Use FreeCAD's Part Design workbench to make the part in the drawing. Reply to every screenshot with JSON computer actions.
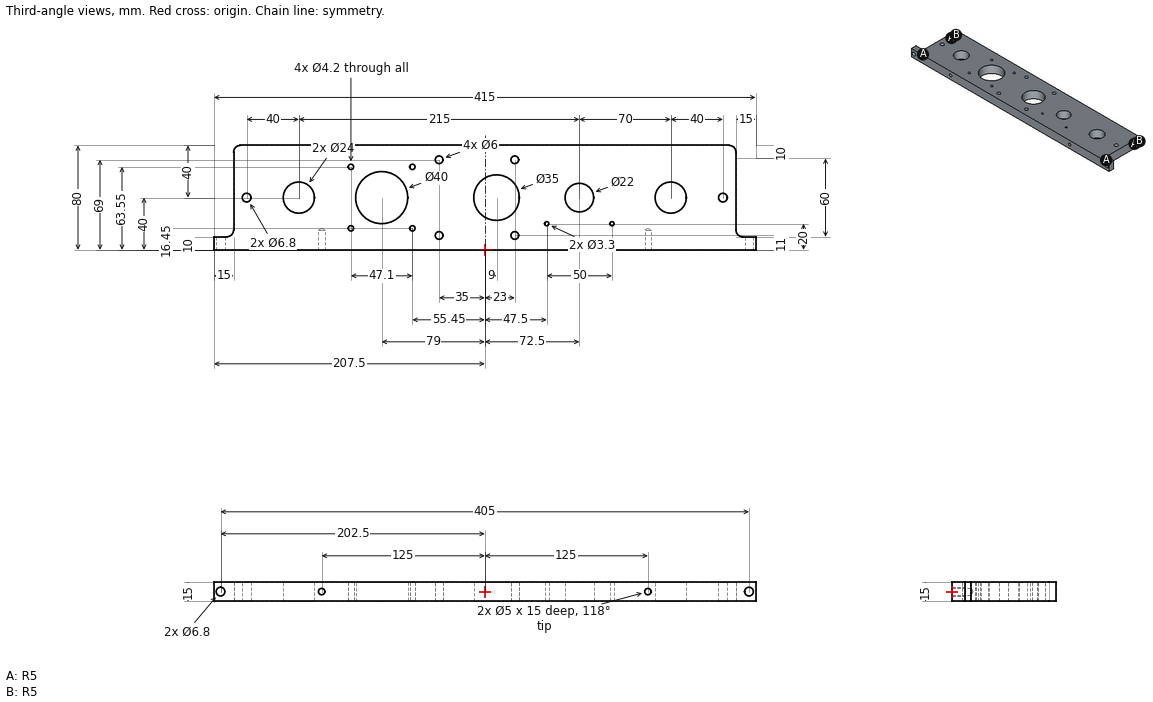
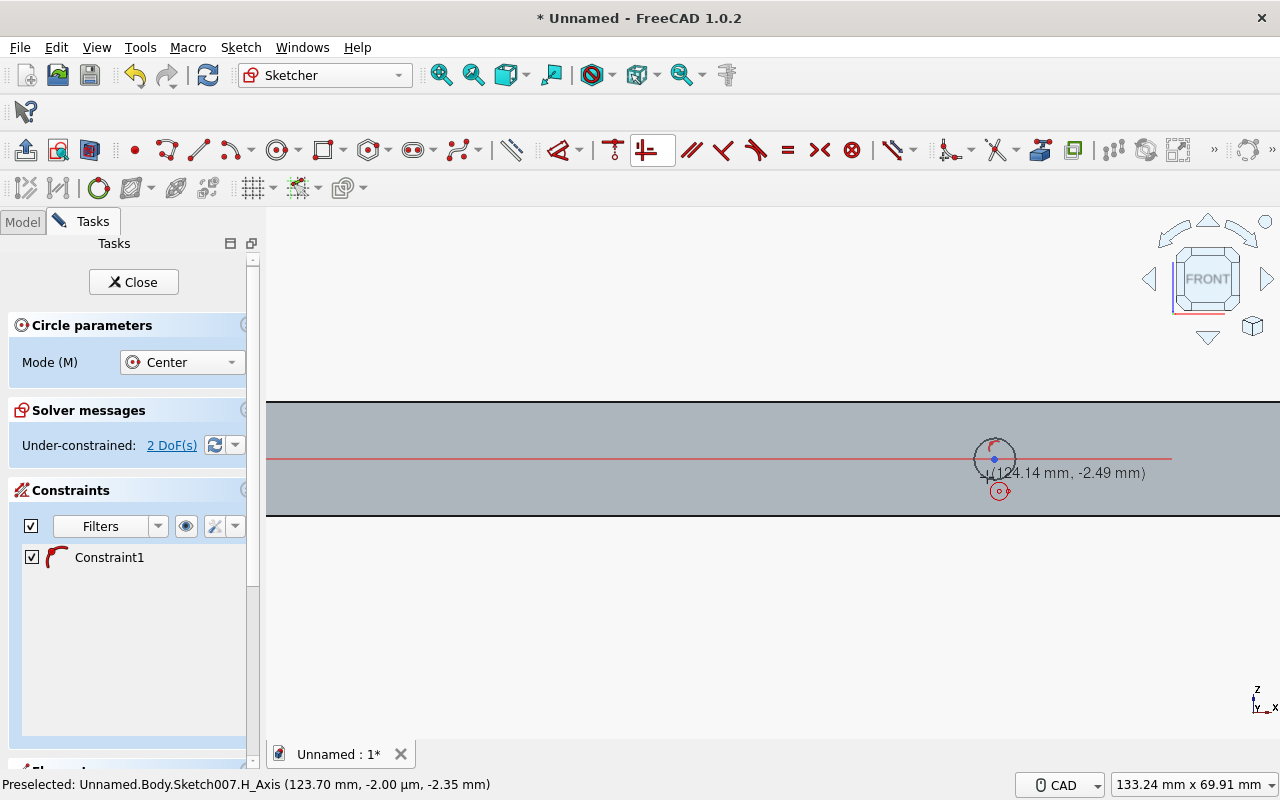
{"action": "scroll", "coordinate": [990, 479], "scroll_direction": "down", "scroll_amount": 6}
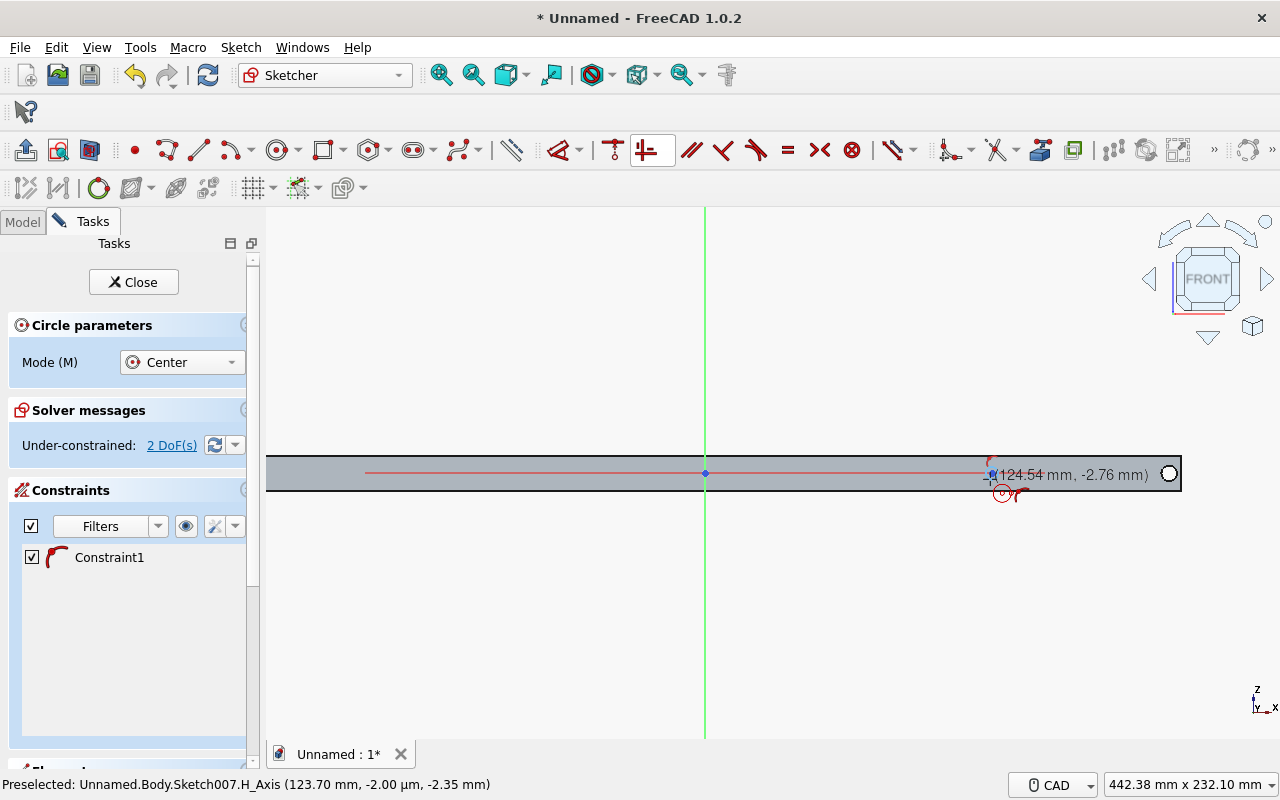
{"action": "scroll", "coordinate": [419, 473], "scroll_direction": "up", "scroll_amount": 7}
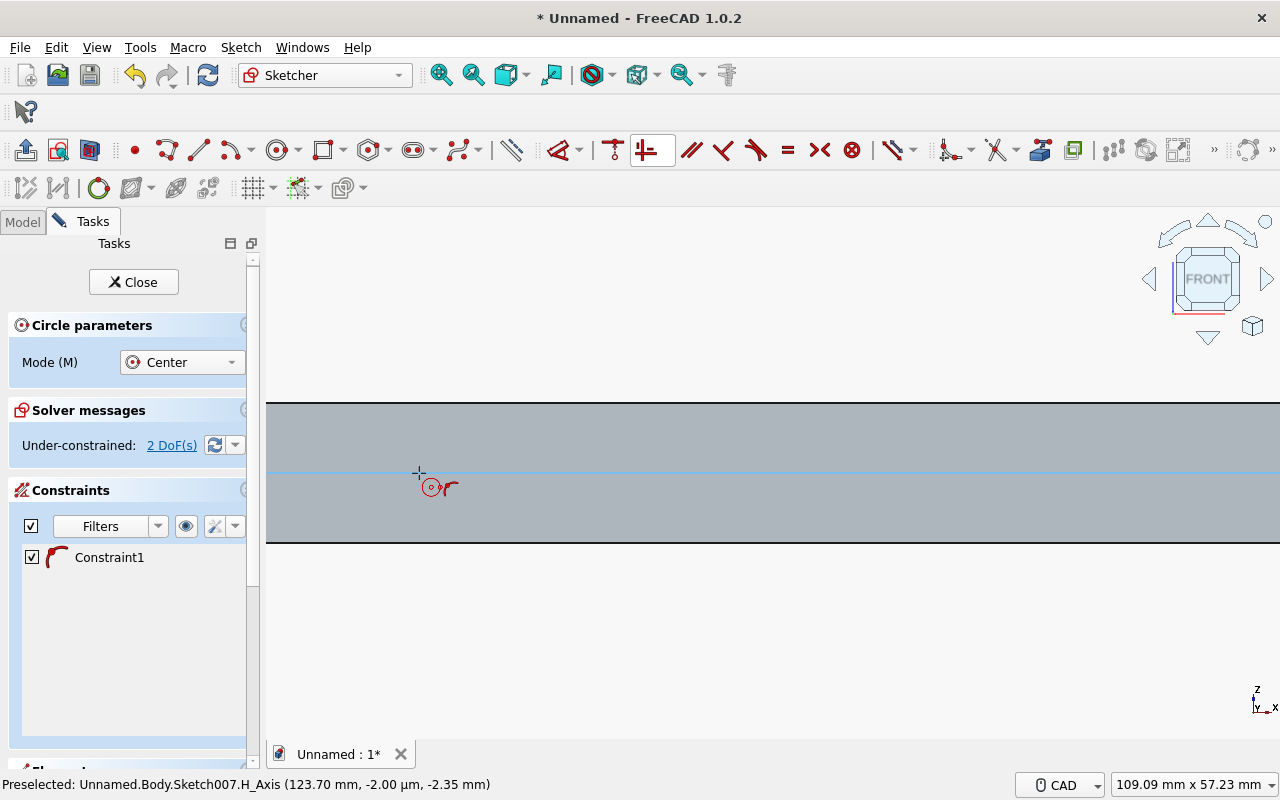
{"action": "scroll", "coordinate": [418, 473], "scroll_direction": "down", "scroll_amount": 7}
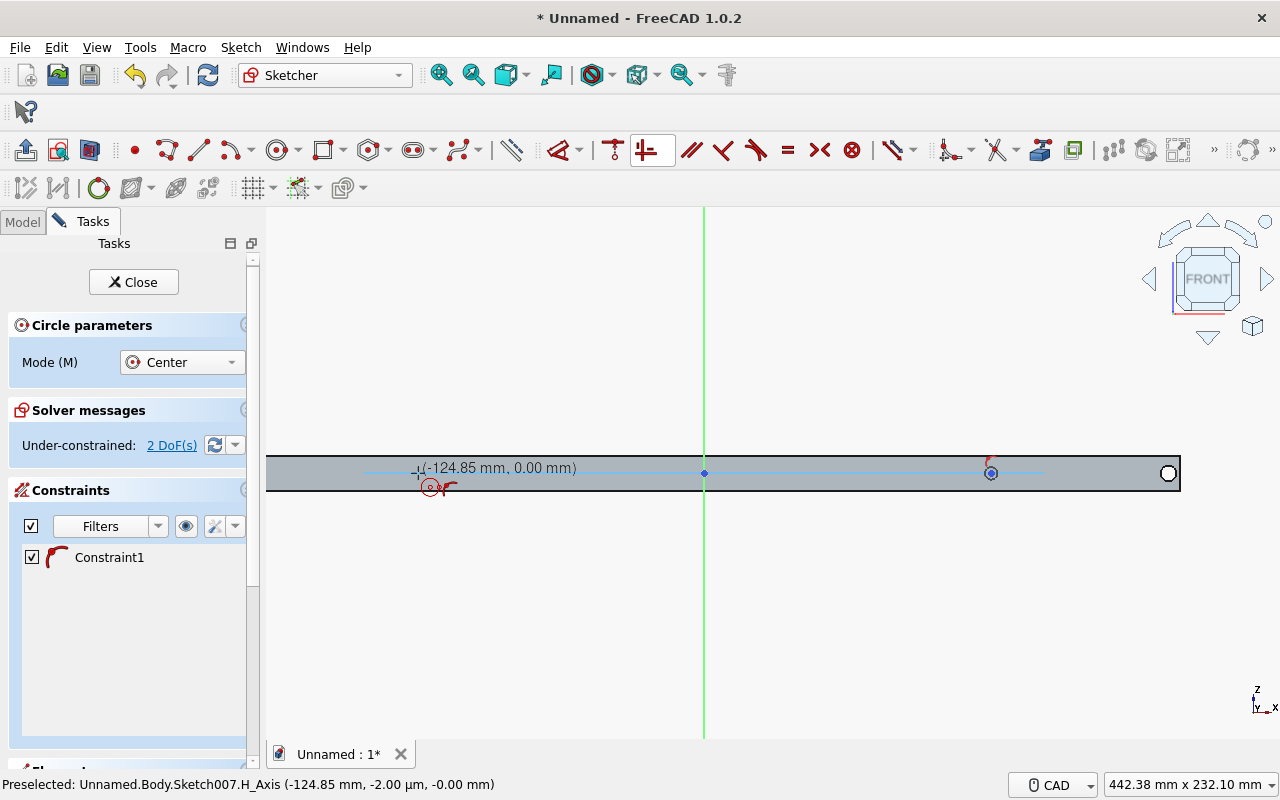
{"action": "left_click", "coordinate": [418, 473]}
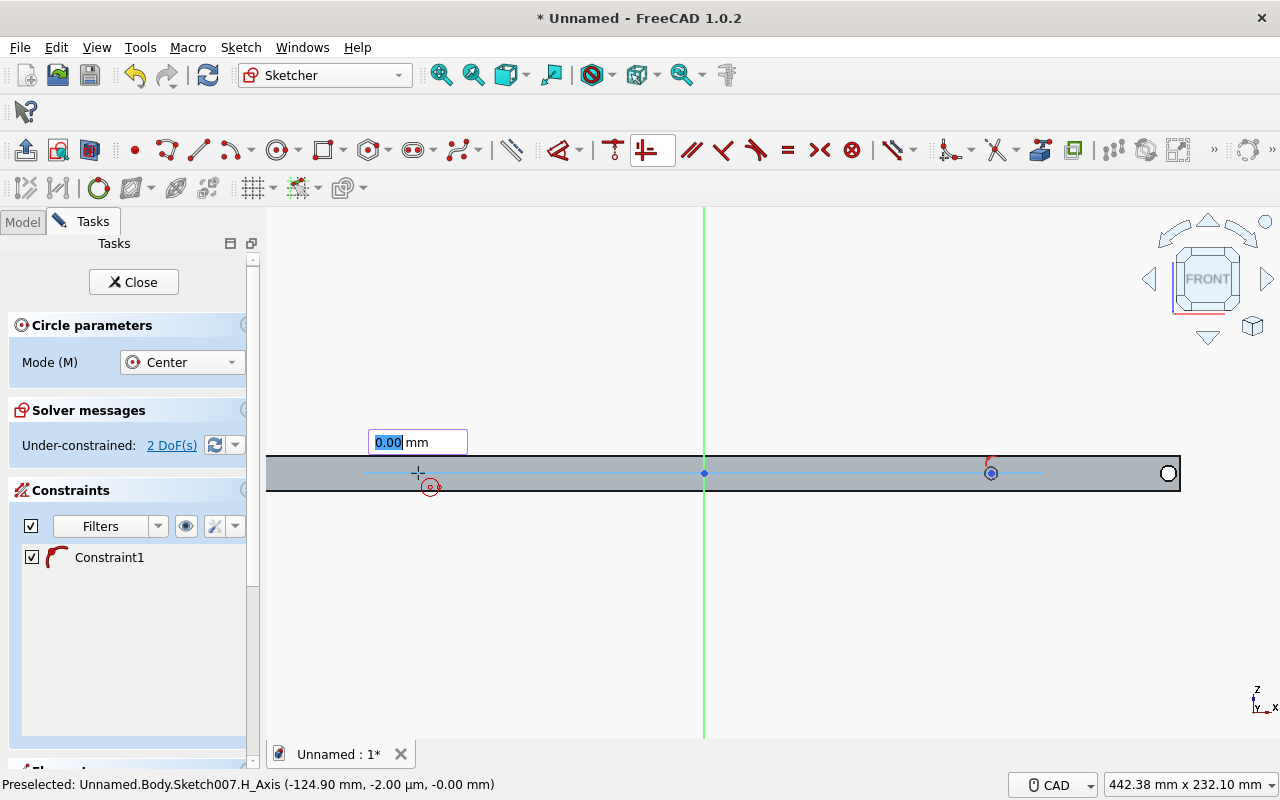
{"action": "scroll", "coordinate": [416, 479], "scroll_direction": "up", "scroll_amount": 6}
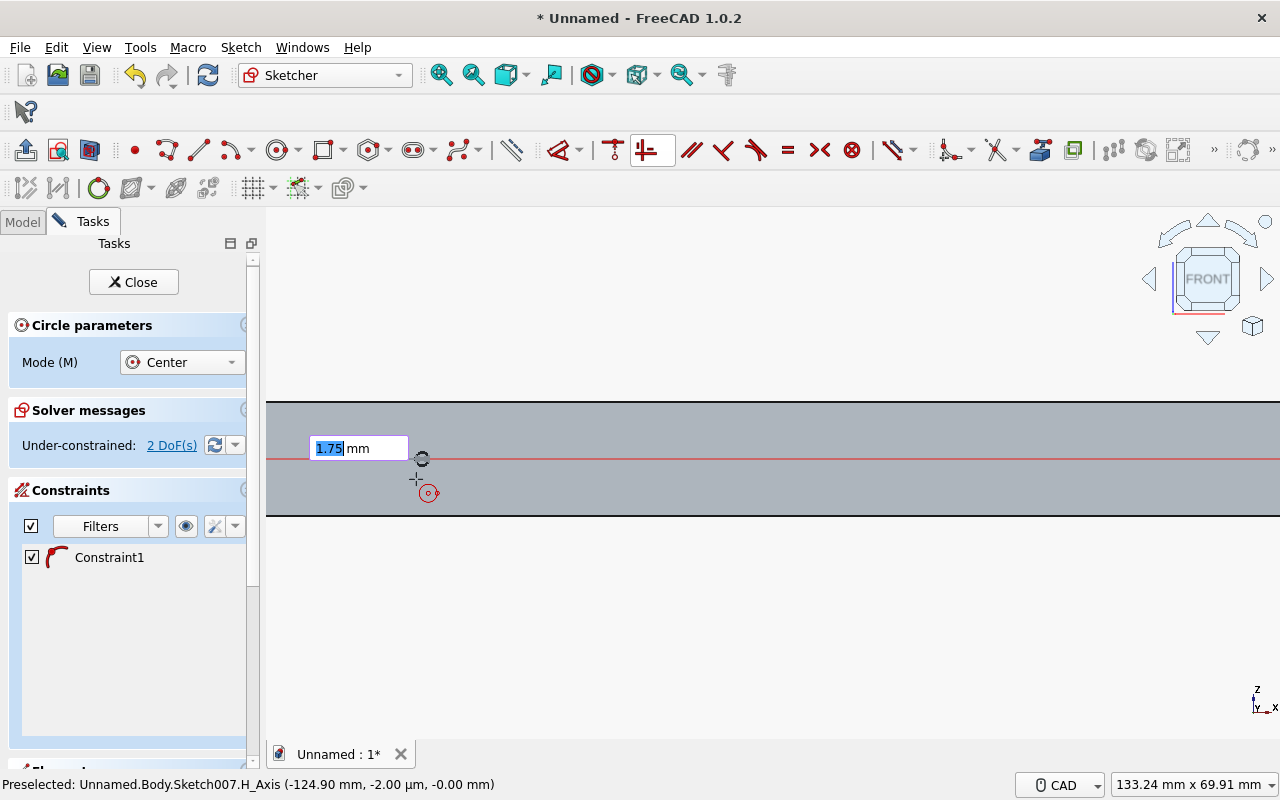
{"action": "left_click", "coordinate": [415, 477]}
{"action": "key", "text": "Escape"}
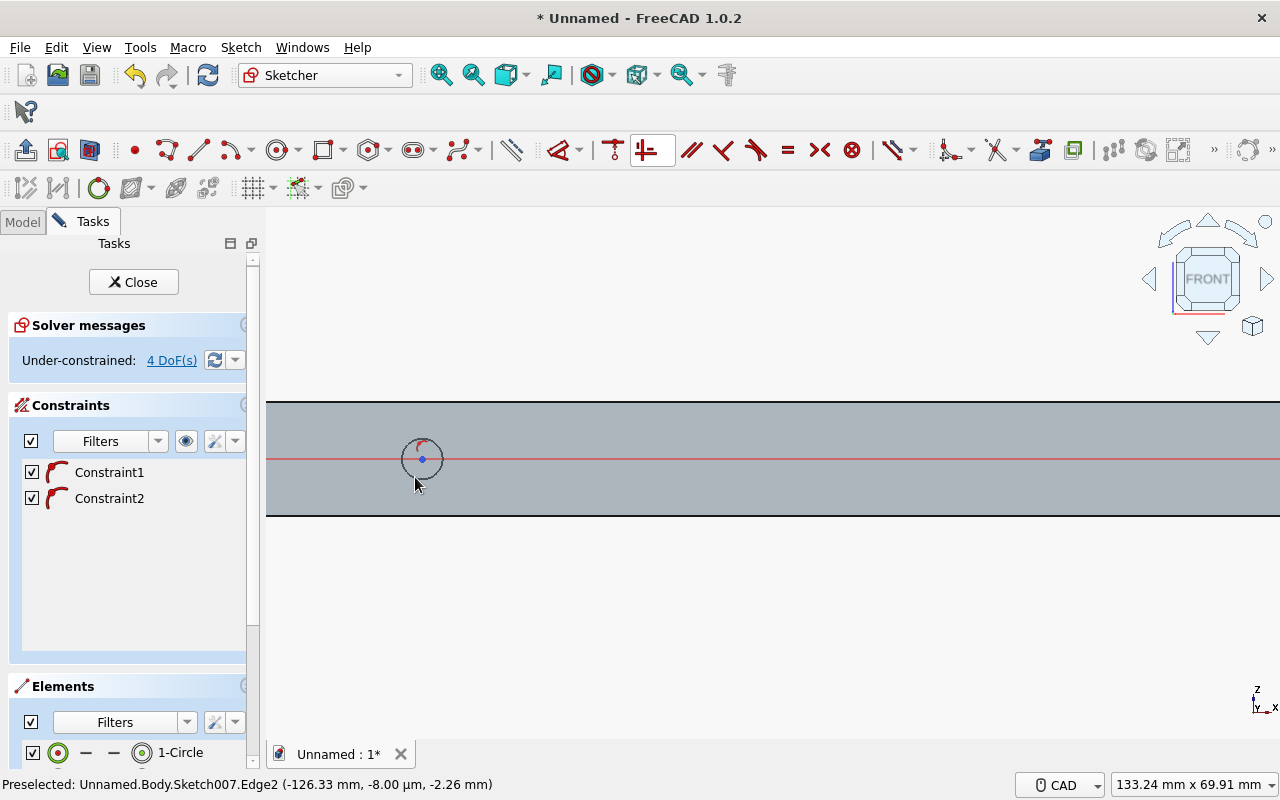
{"action": "scroll", "coordinate": [416, 479], "scroll_direction": "down", "scroll_amount": 6}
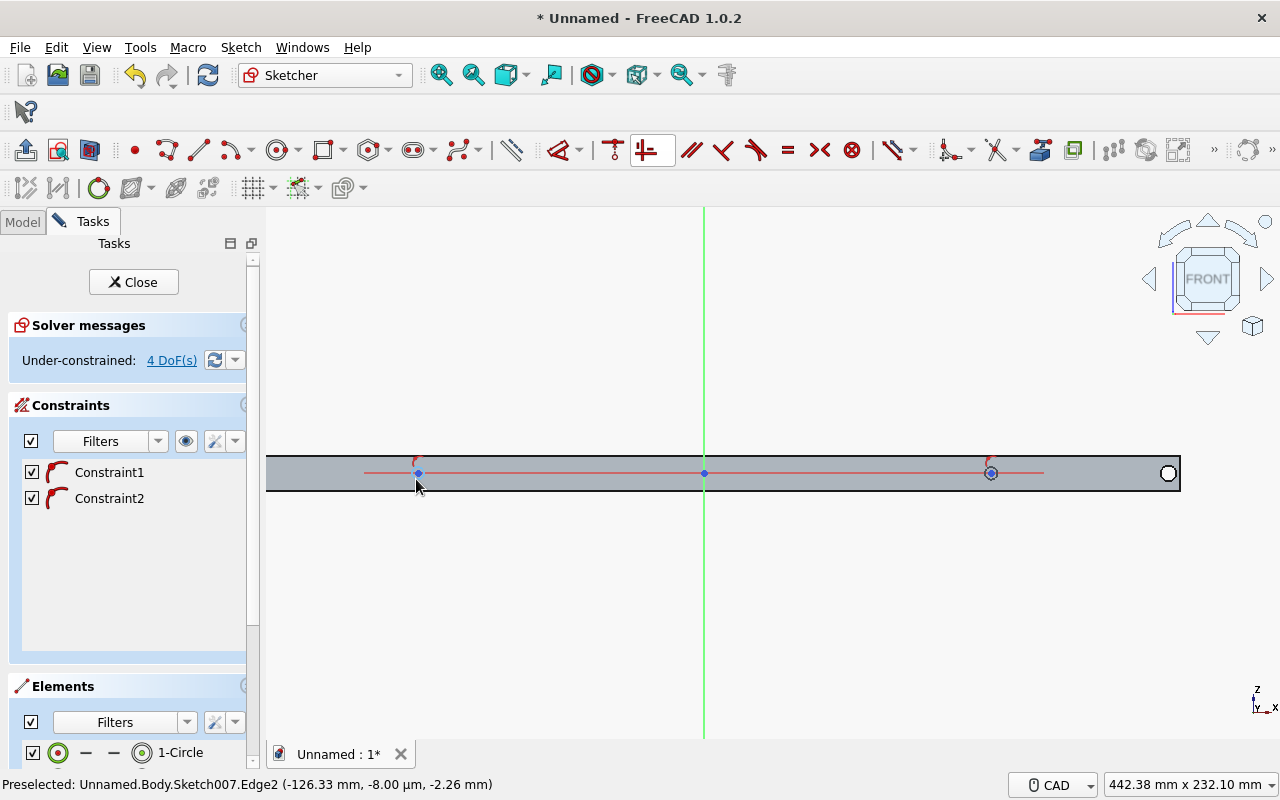
{"action": "scroll", "coordinate": [996, 469], "scroll_direction": "up", "scroll_amount": 6}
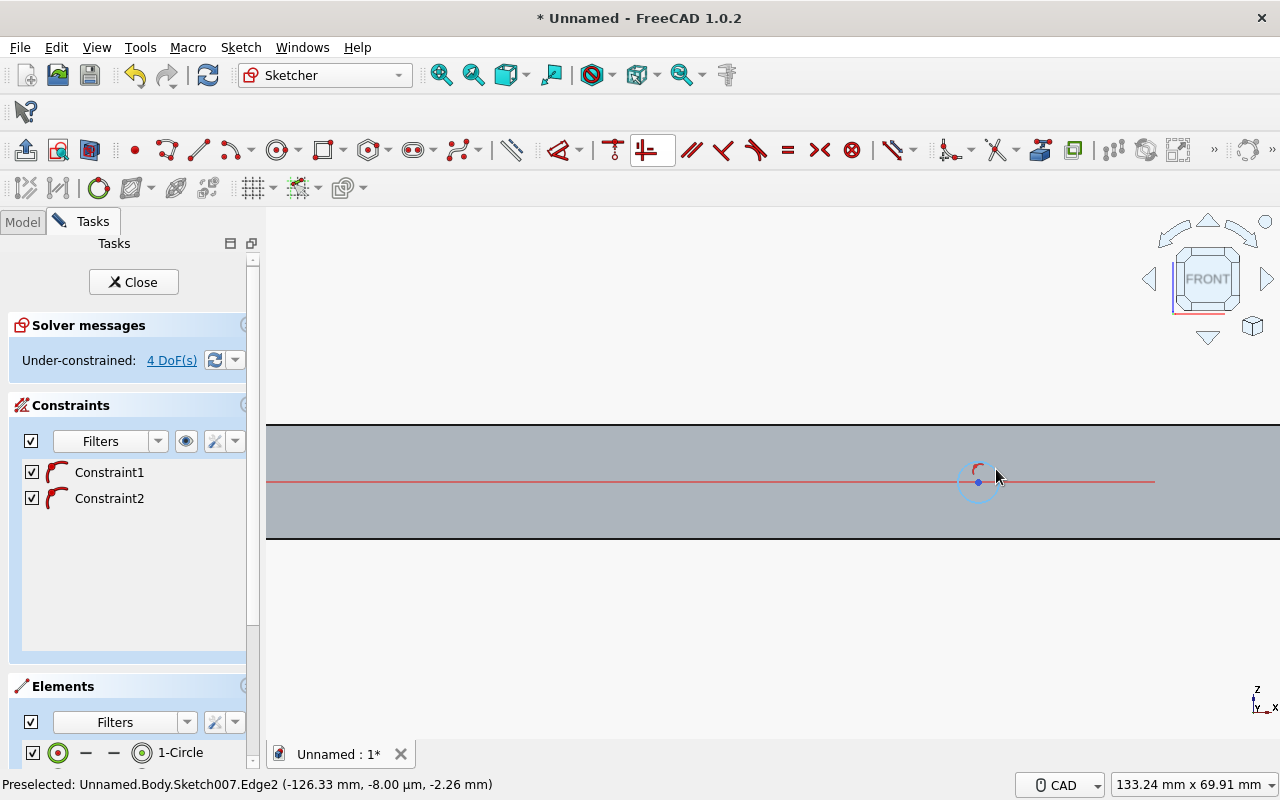
{"action": "left_click", "coordinate": [993, 468]}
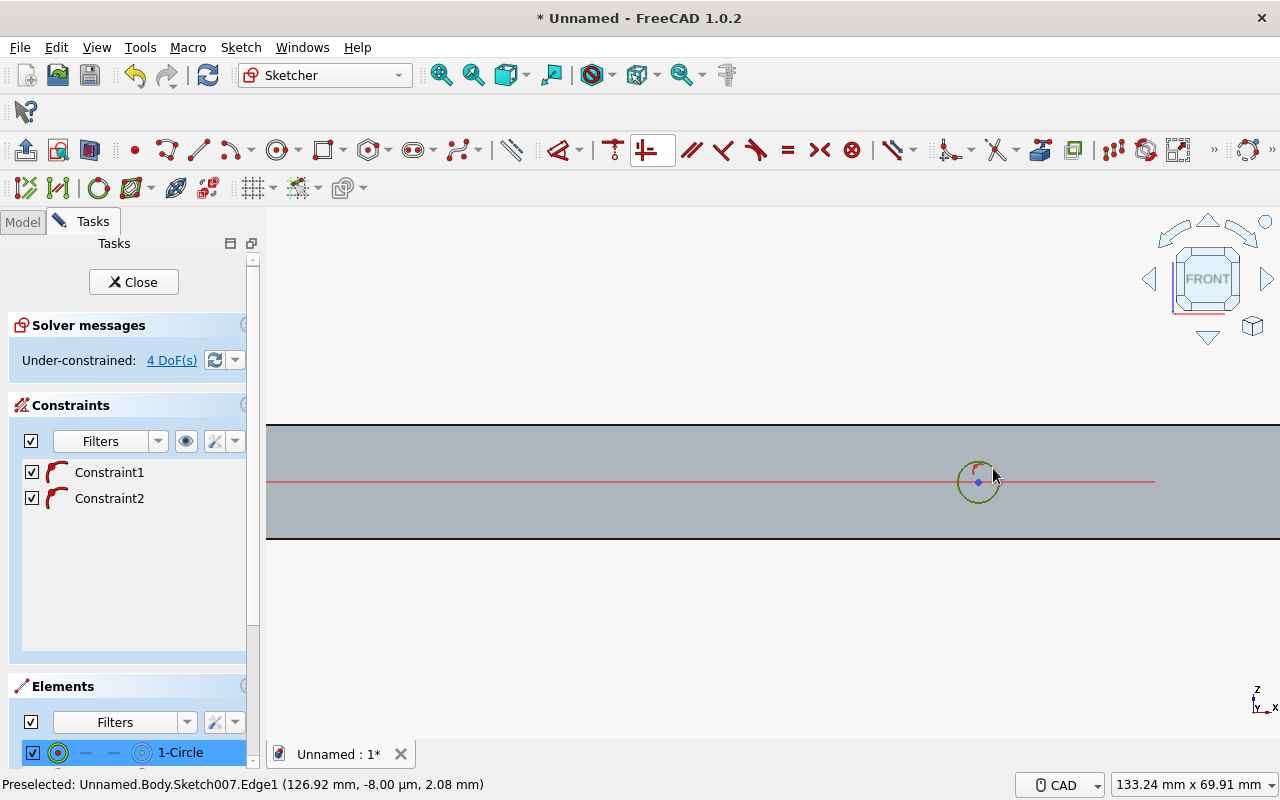
{"action": "scroll", "coordinate": [997, 469], "scroll_direction": "down", "scroll_amount": 6}